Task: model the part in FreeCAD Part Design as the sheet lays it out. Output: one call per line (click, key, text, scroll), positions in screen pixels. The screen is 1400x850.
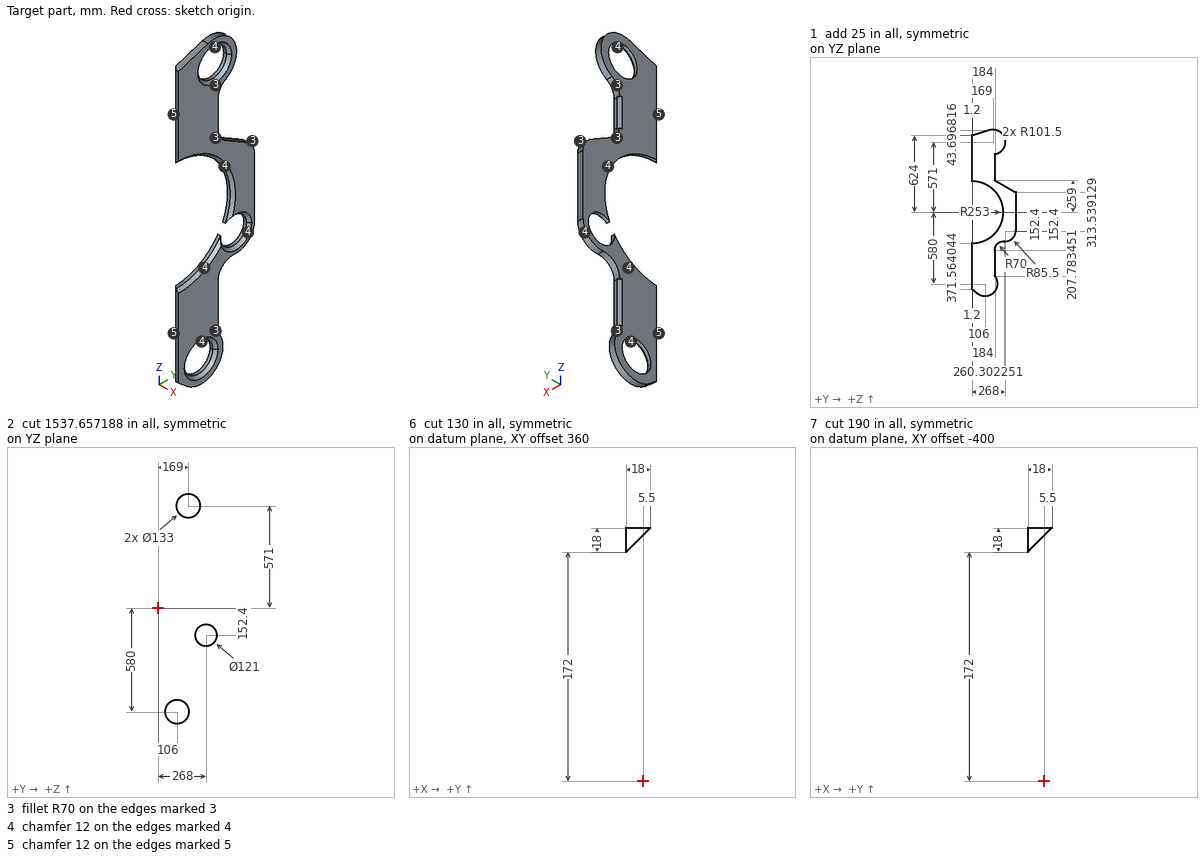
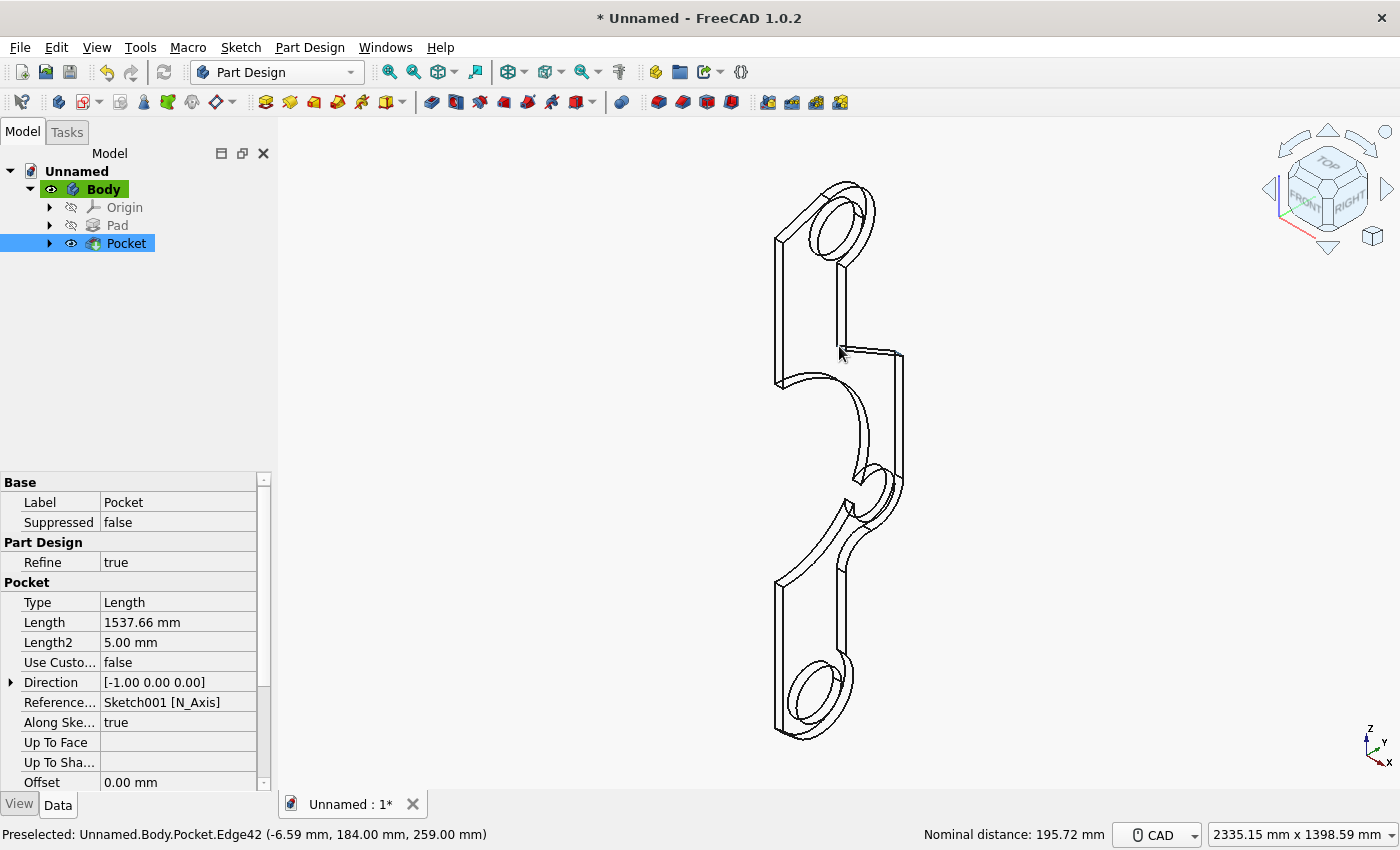
click(839, 649, ctrl)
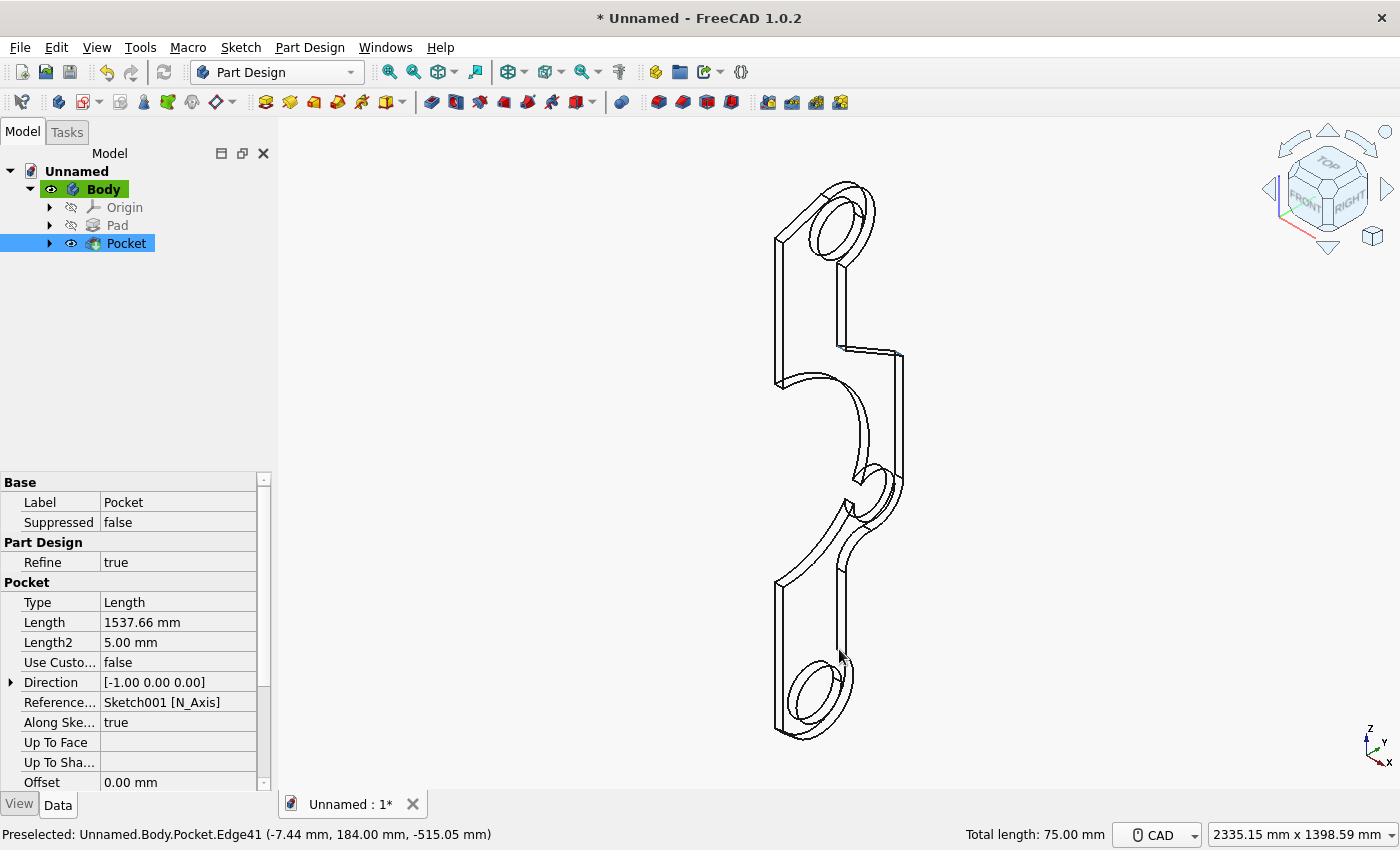
scroll(841, 264, up, 7)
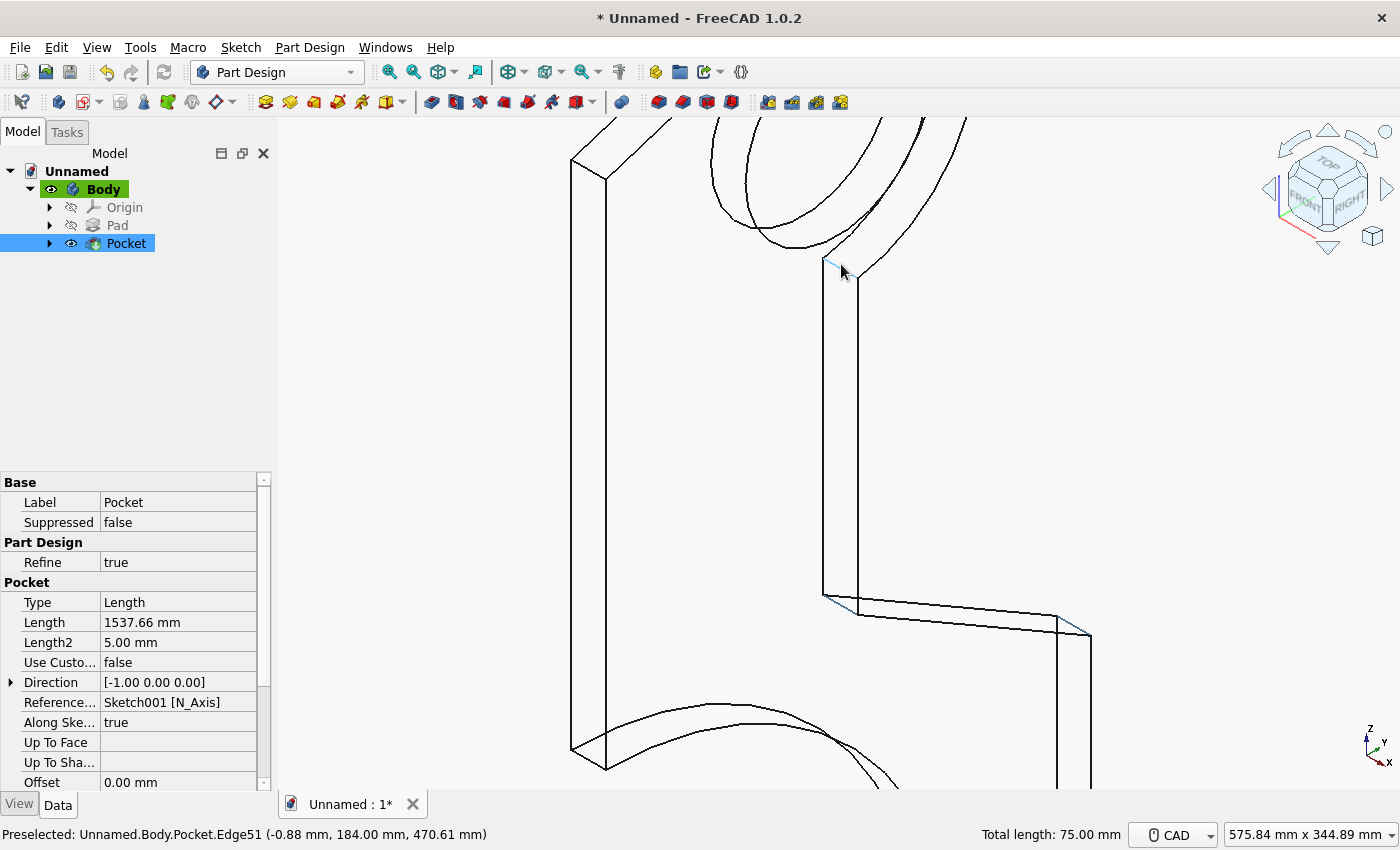
click(841, 267, ctrl)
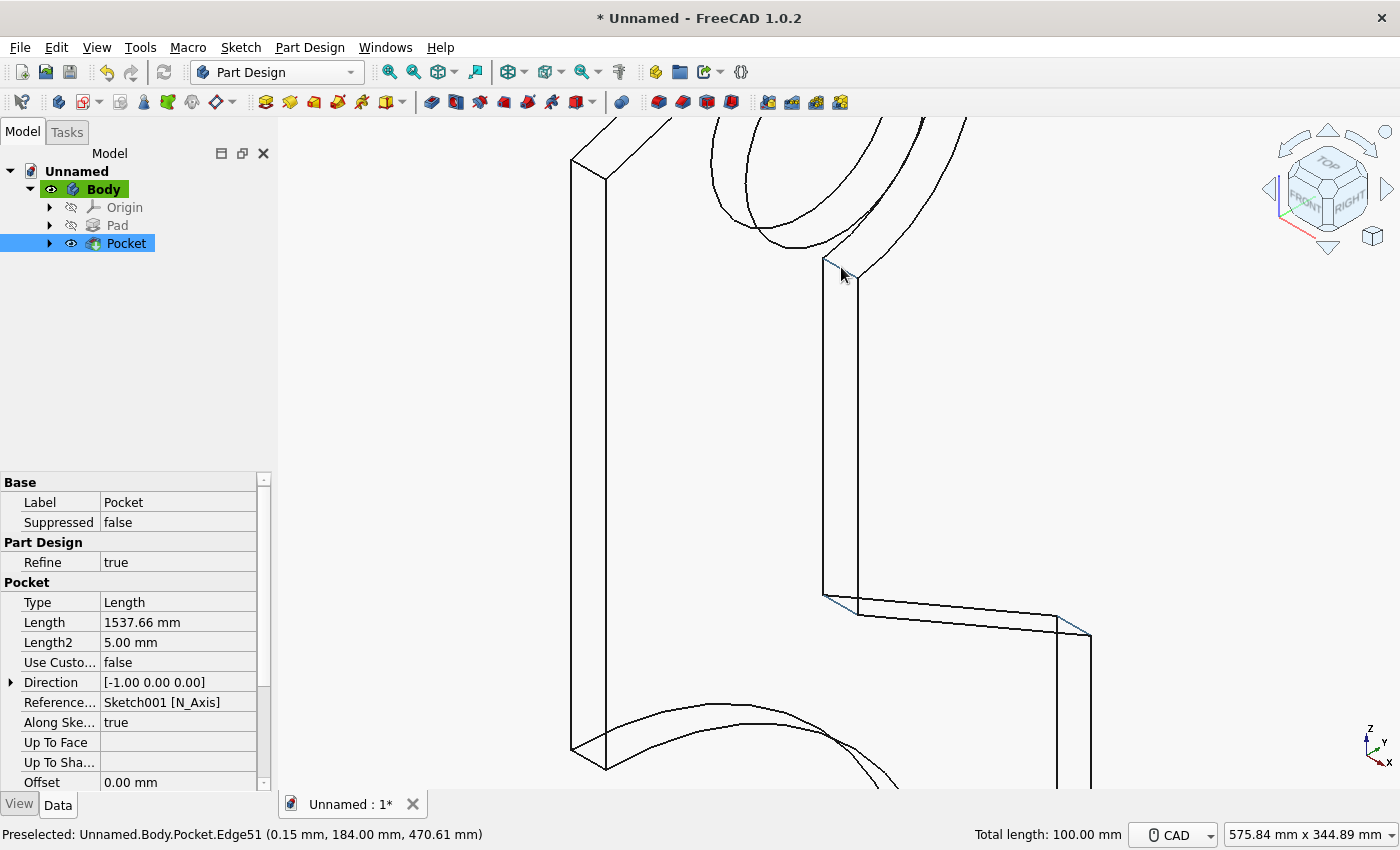
key(v)
key(1)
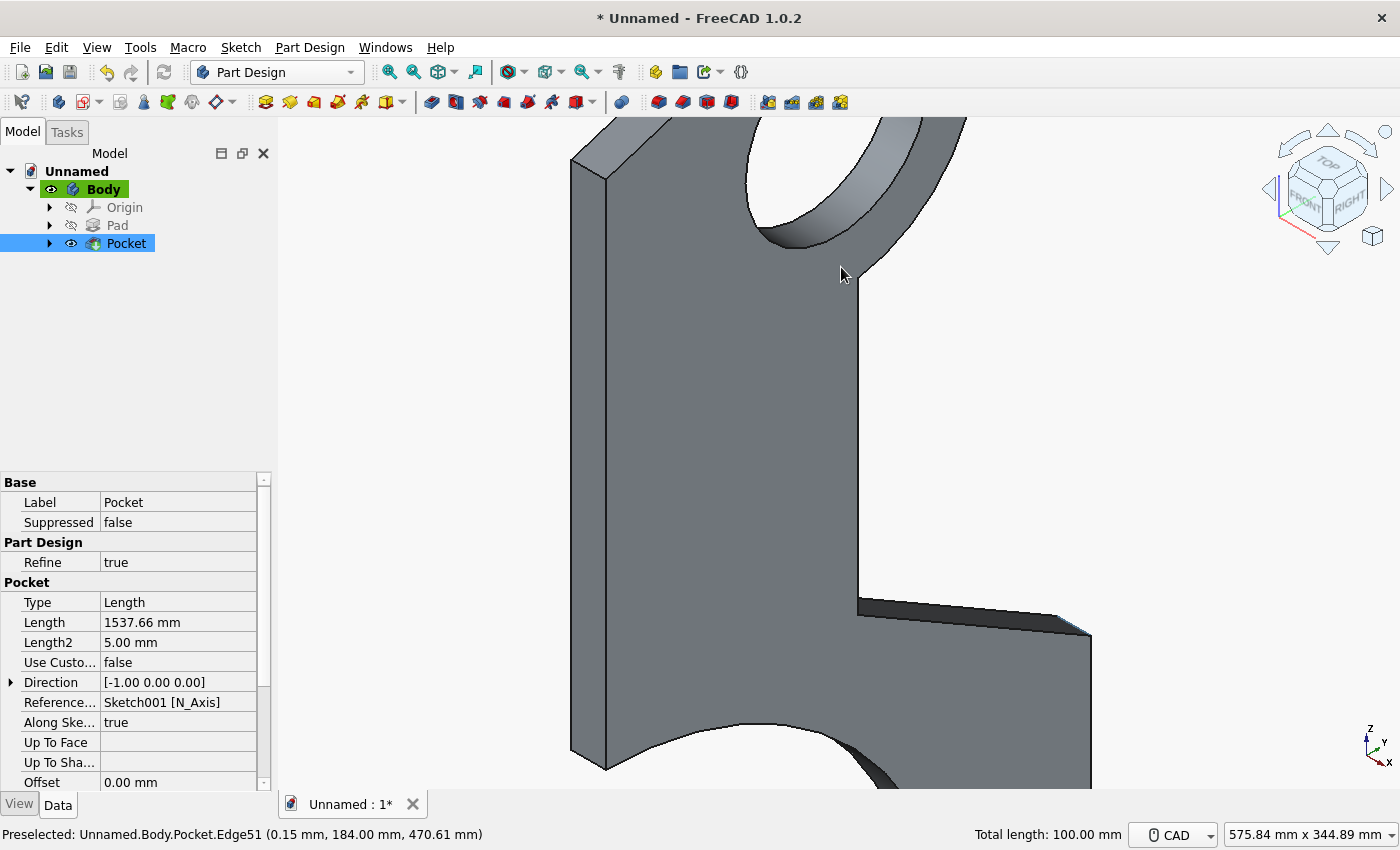
click(660, 102)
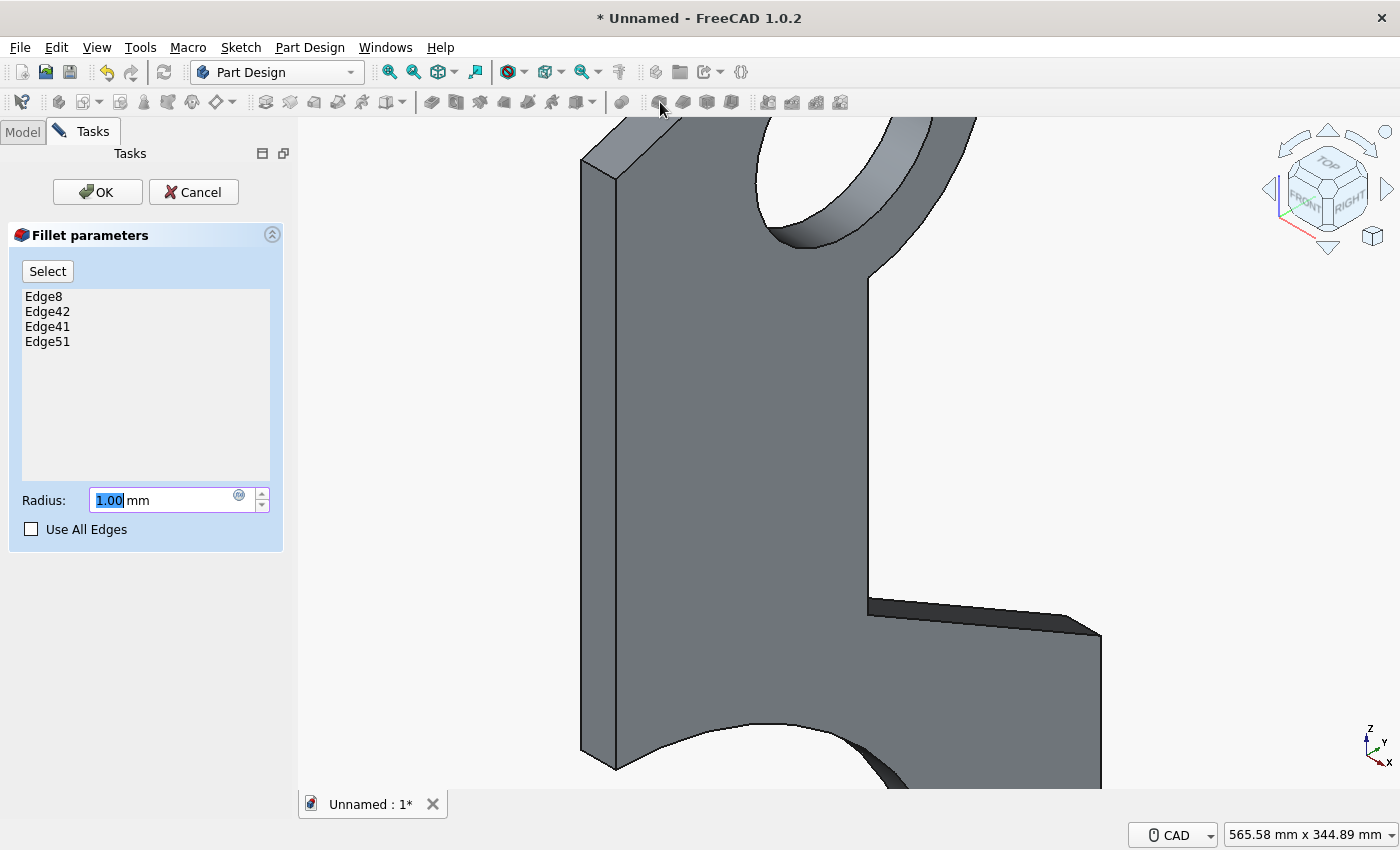
text(70)
key(Tab)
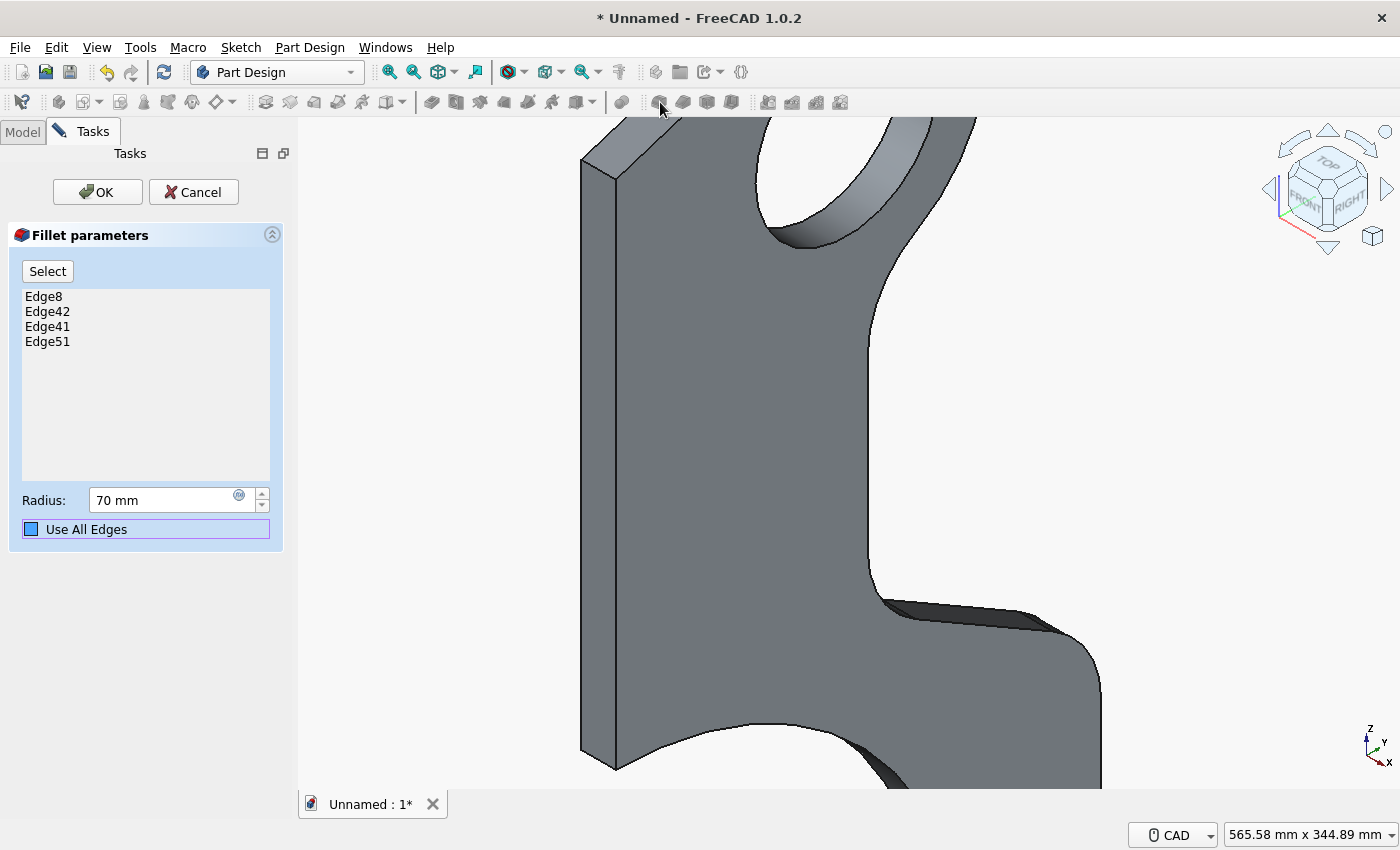
click(98, 192)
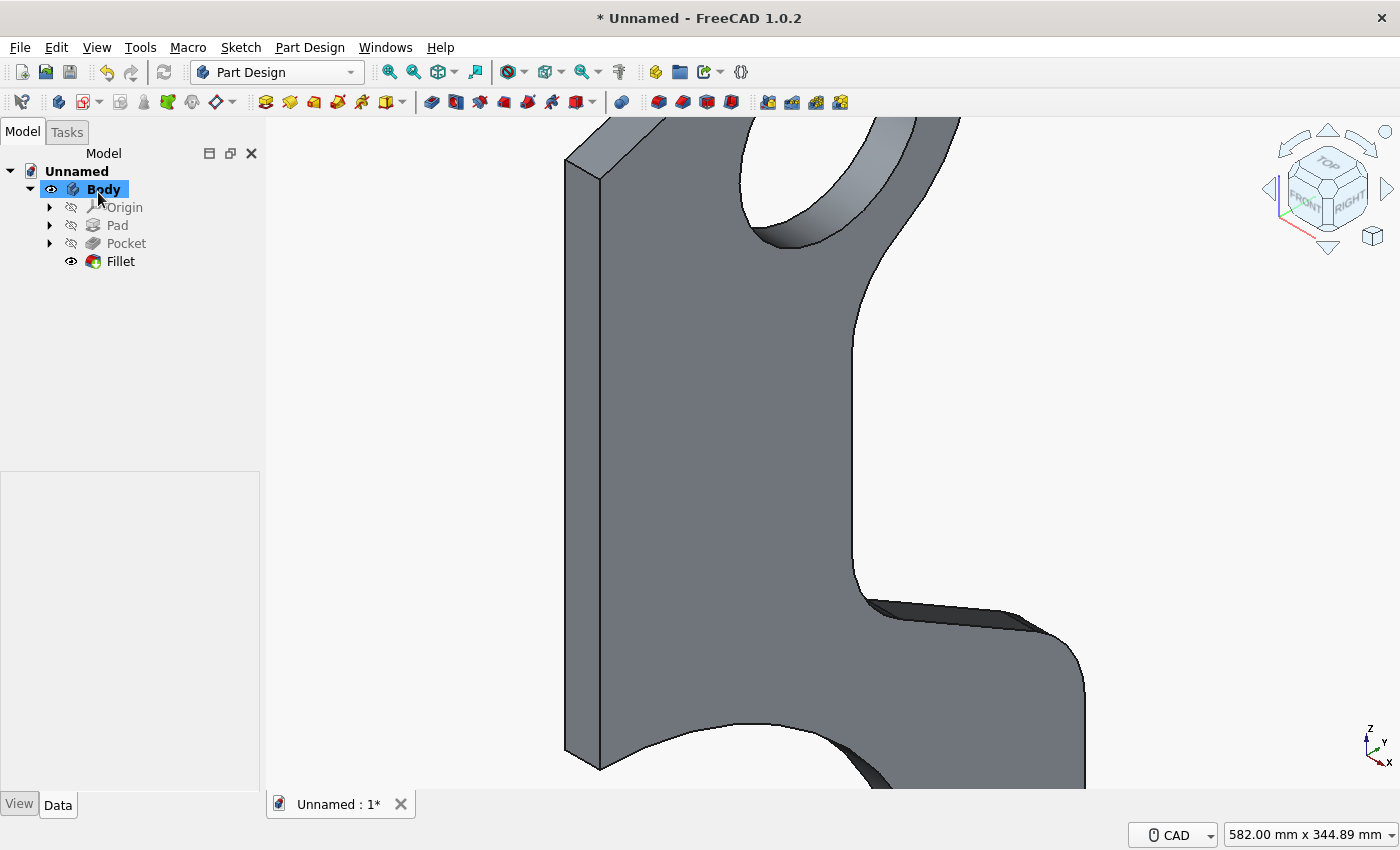
key(v)
key(f)